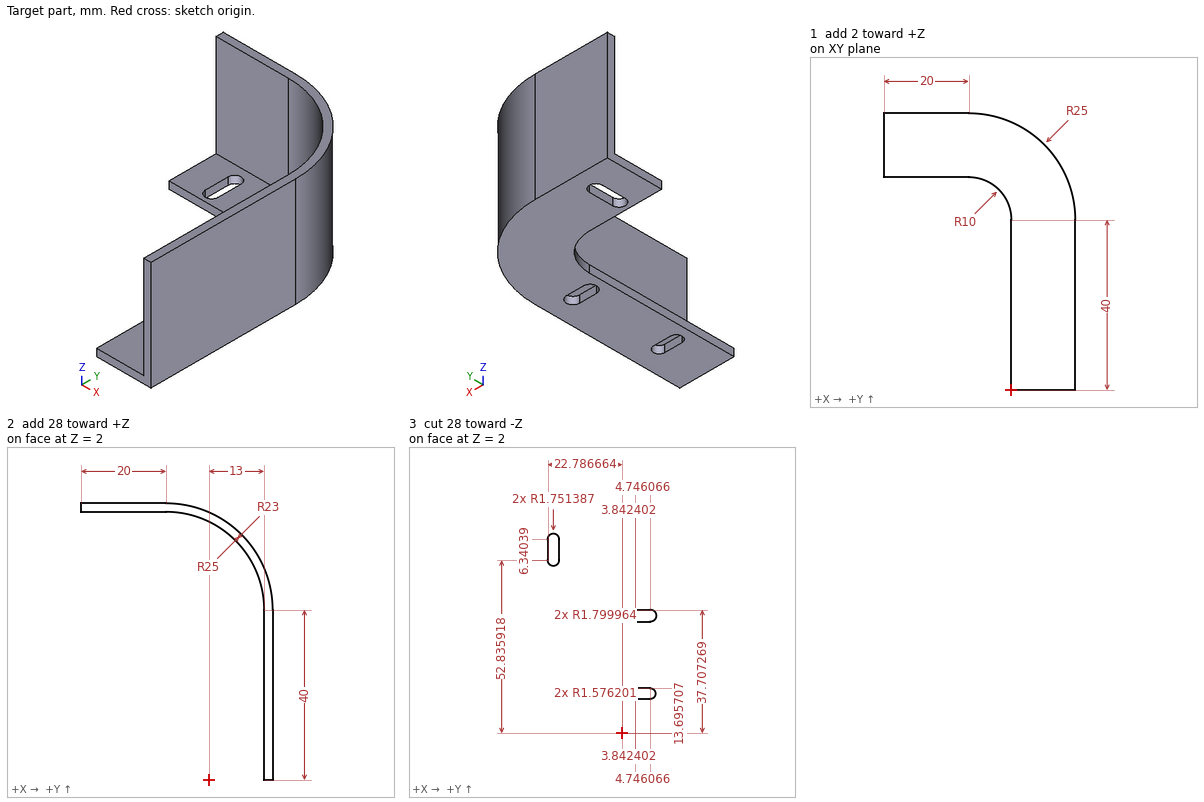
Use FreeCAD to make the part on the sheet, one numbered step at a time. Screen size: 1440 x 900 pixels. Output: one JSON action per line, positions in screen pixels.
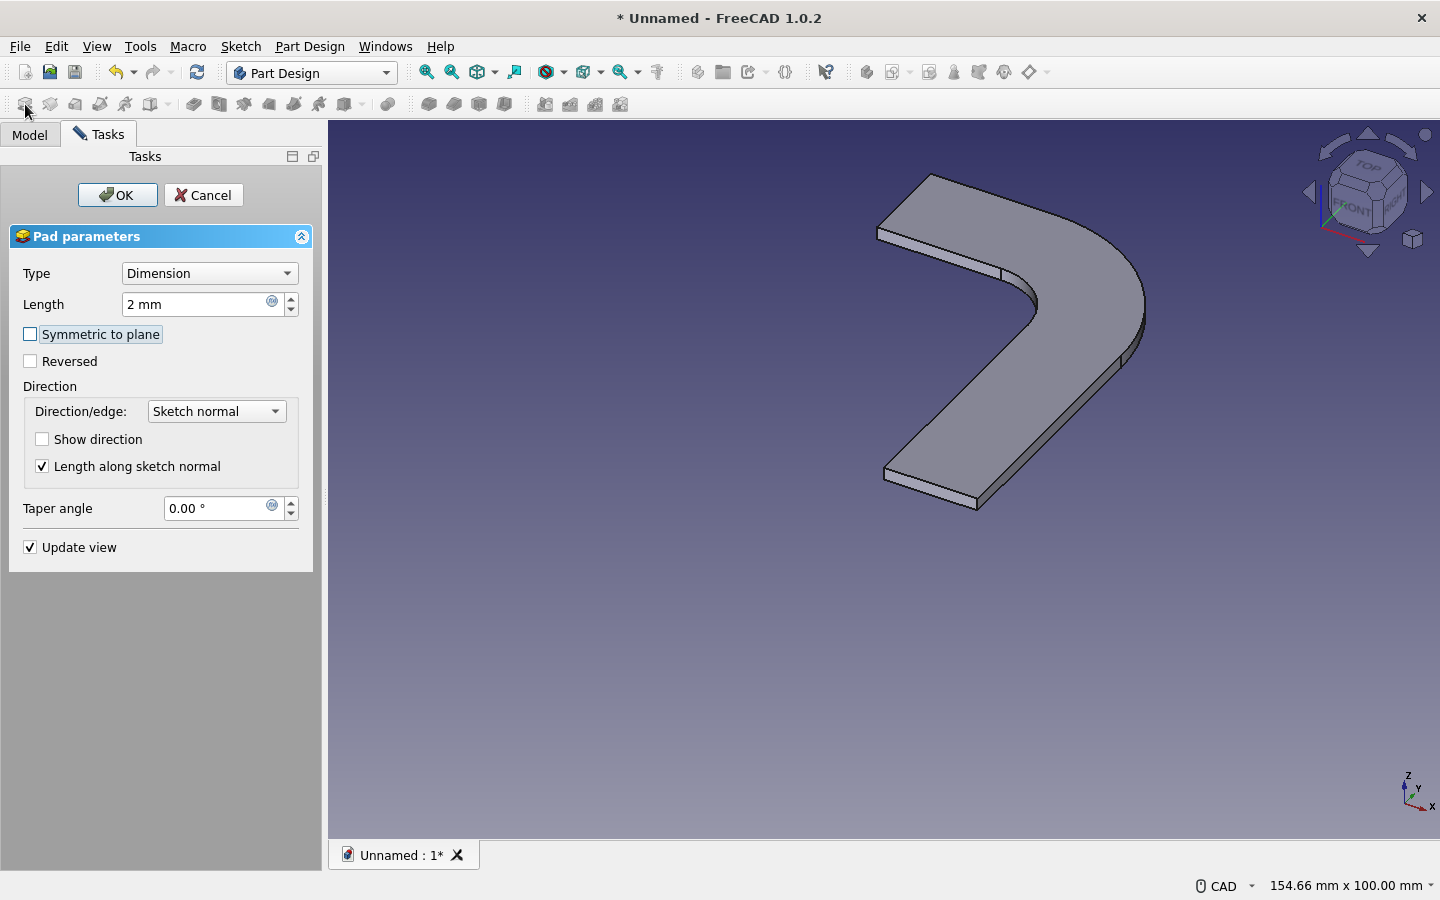
{"action": "left_click", "coordinate": [118, 195]}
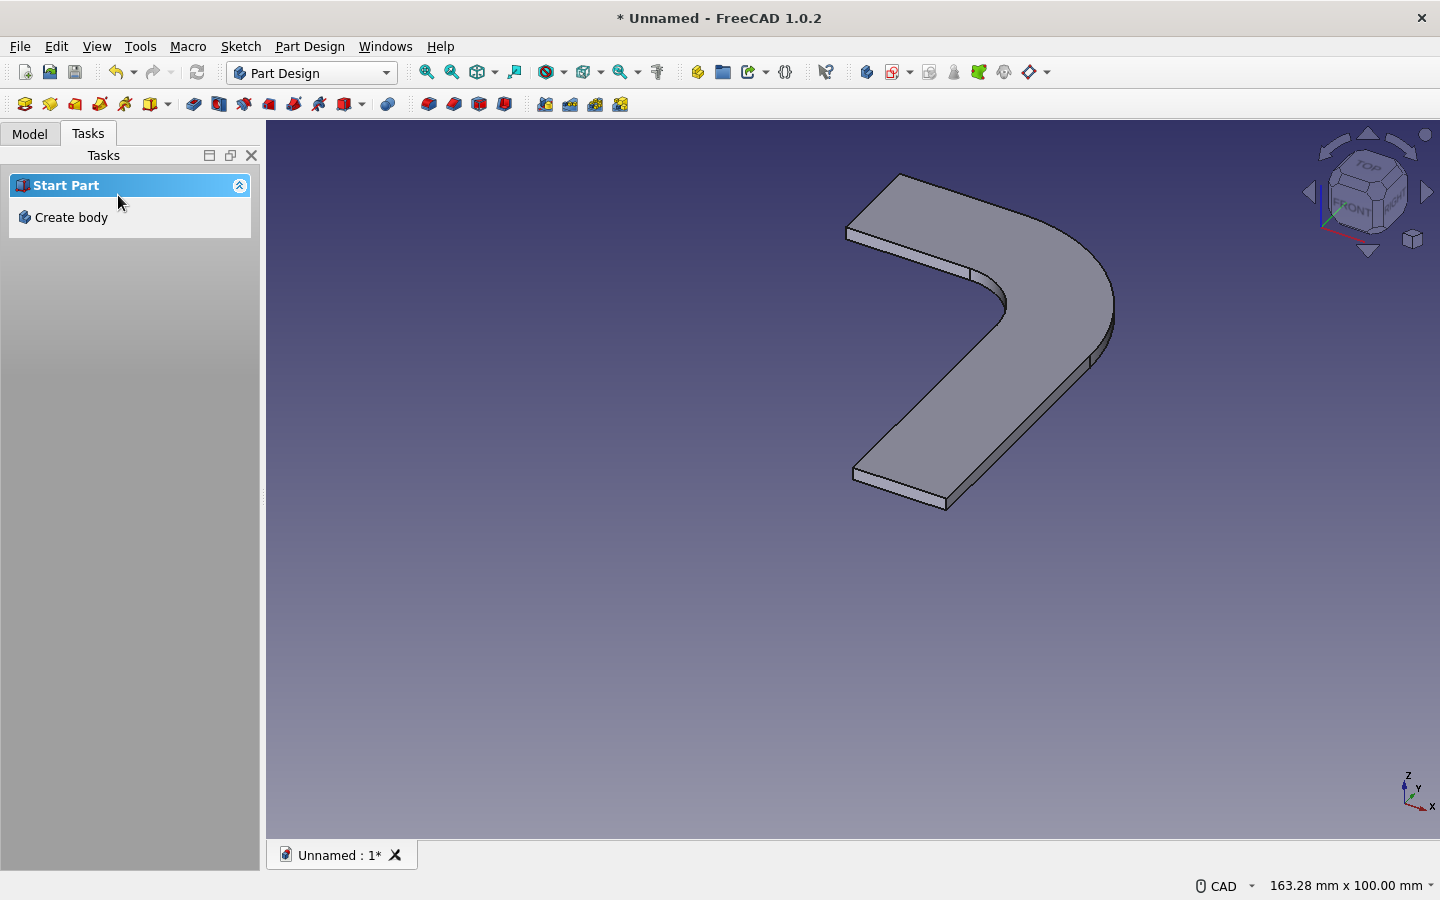
{"action": "left_click", "coordinate": [1070, 295]}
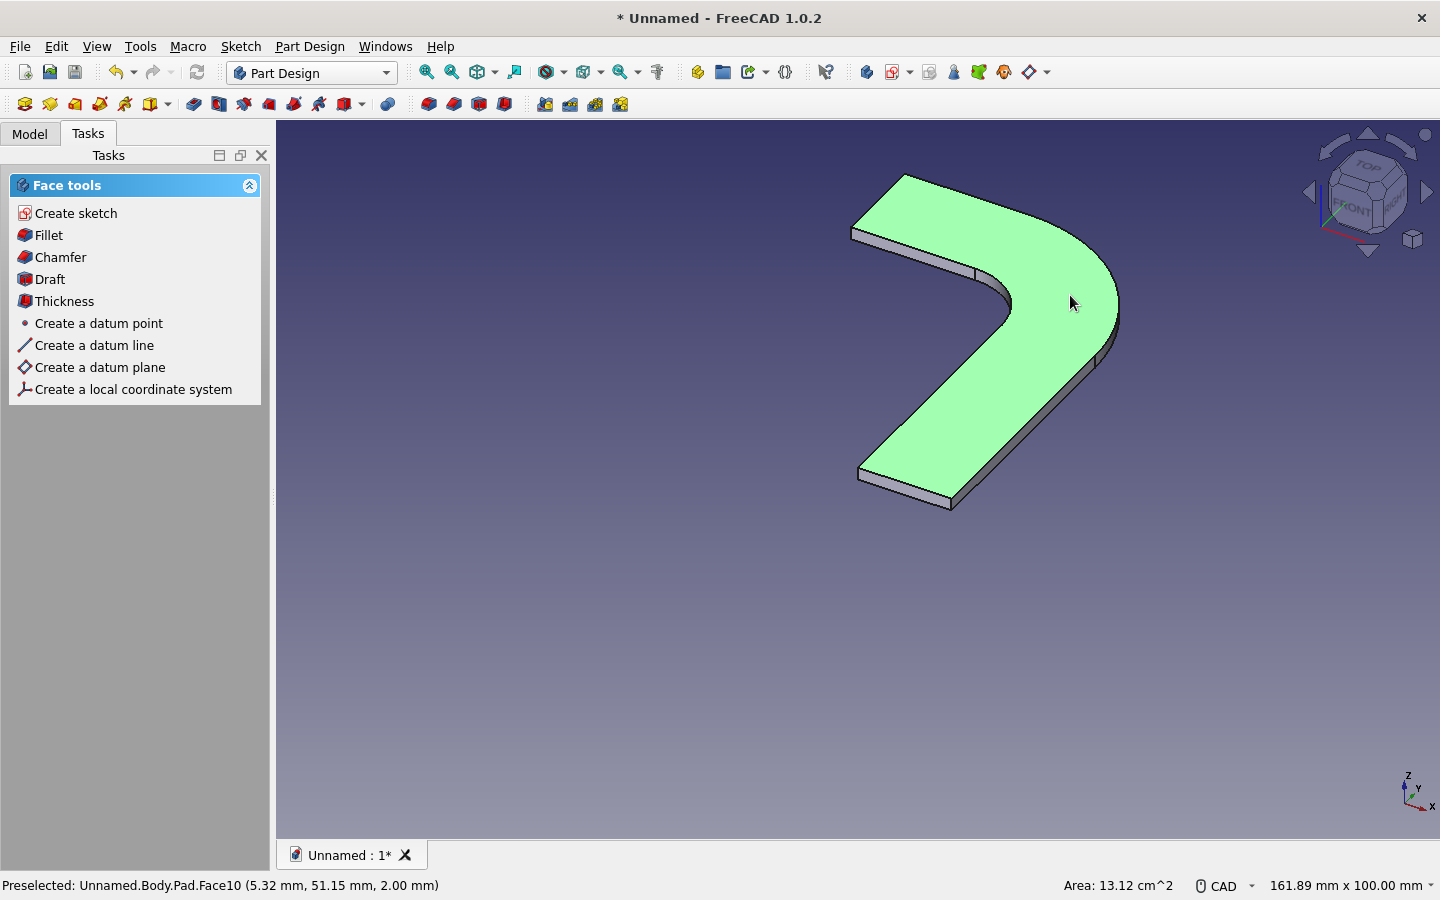
{"action": "left_click", "coordinate": [892, 72]}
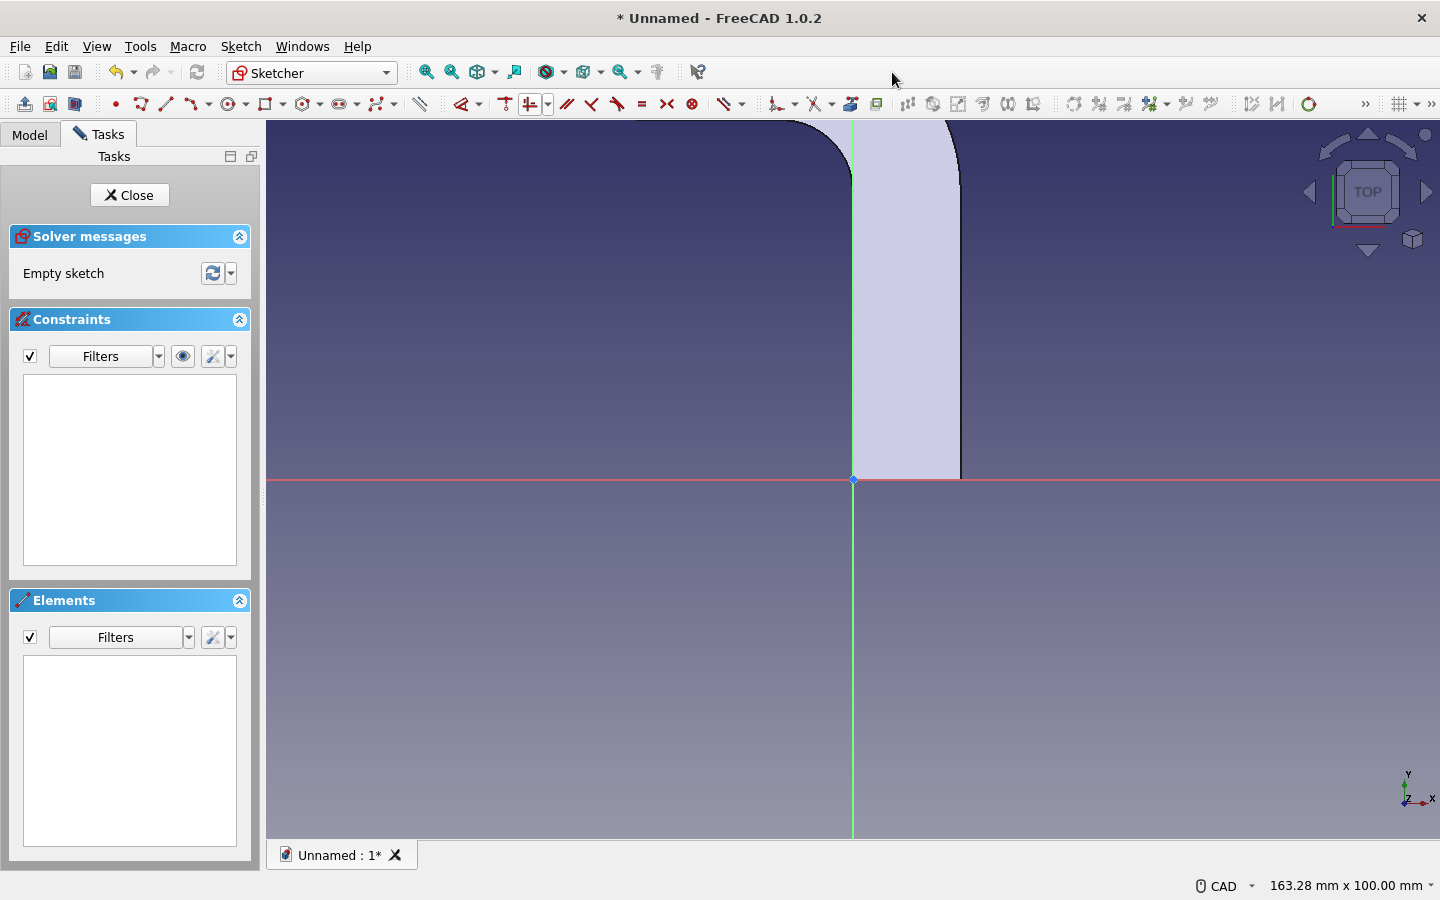
{"action": "scroll", "coordinate": [755, 811], "scroll_direction": "down", "scroll_amount": 2}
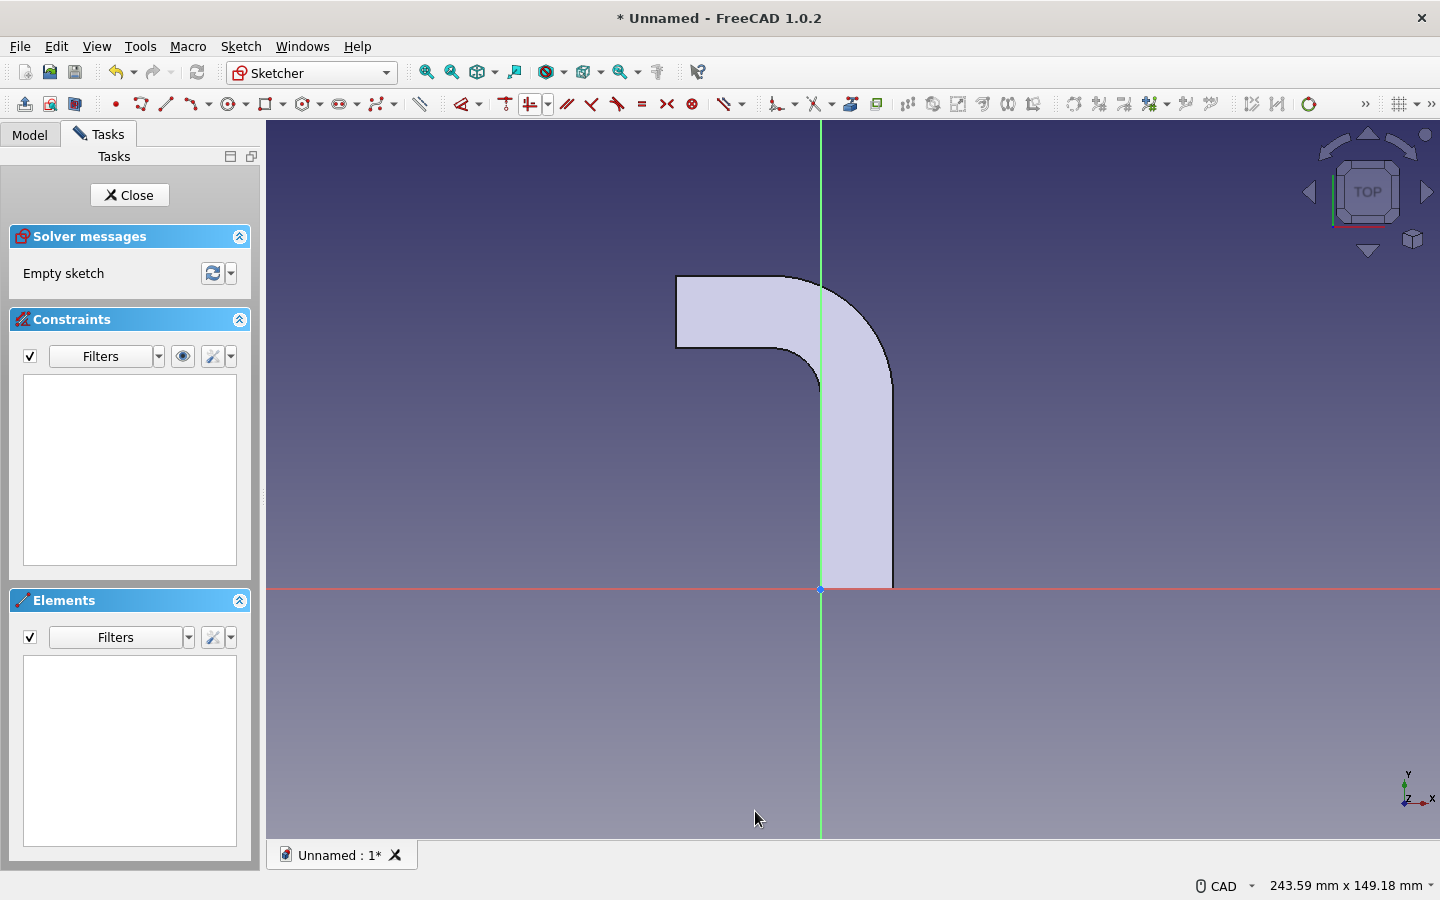
{"action": "scroll", "coordinate": [785, 337], "scroll_direction": "up", "scroll_amount": 2}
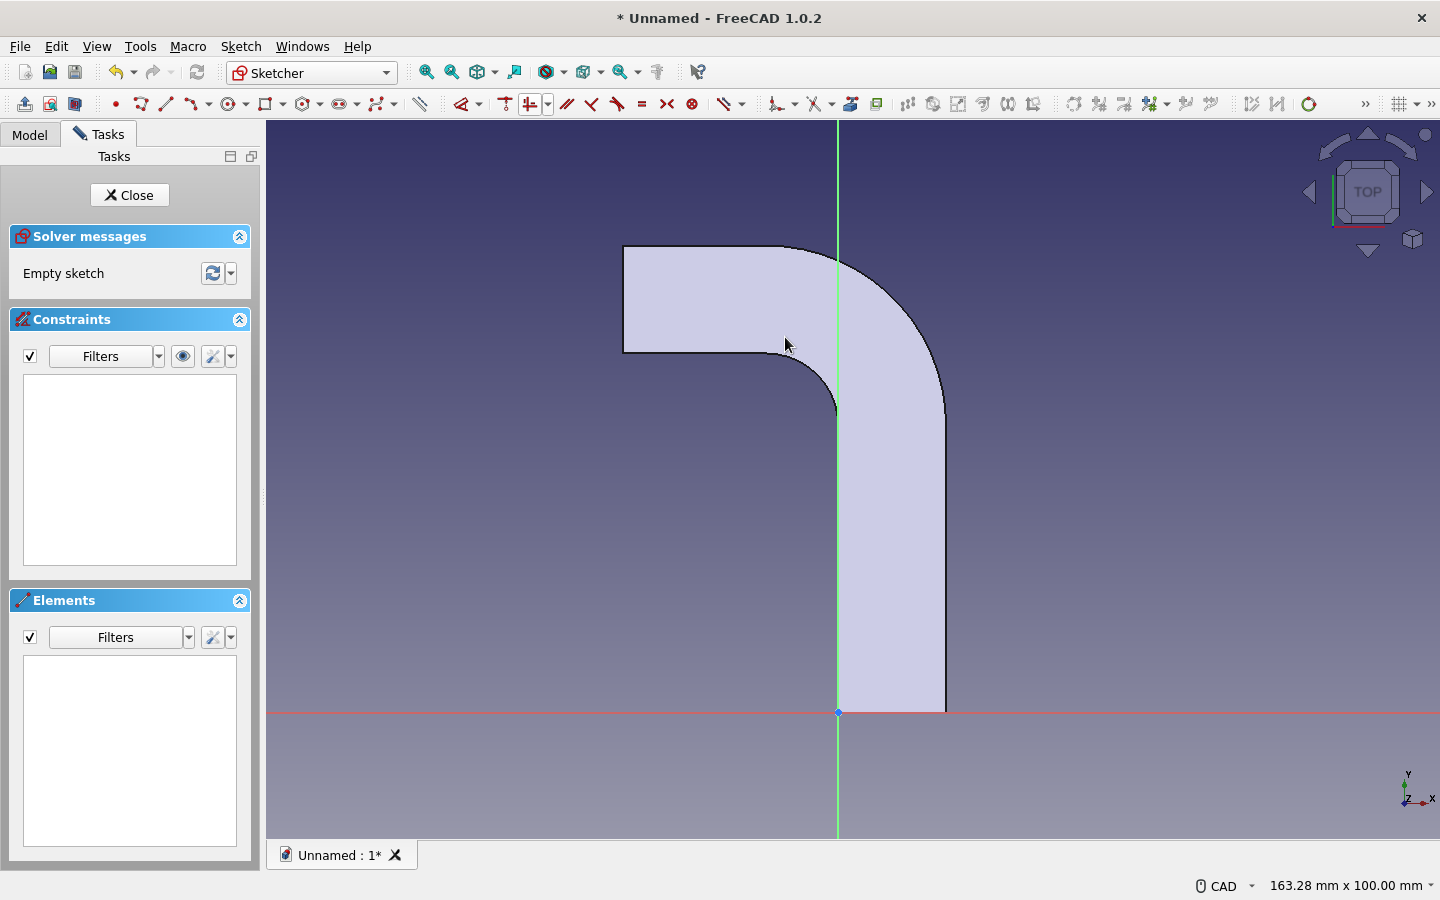
{"action": "left_click", "coordinate": [141, 104]}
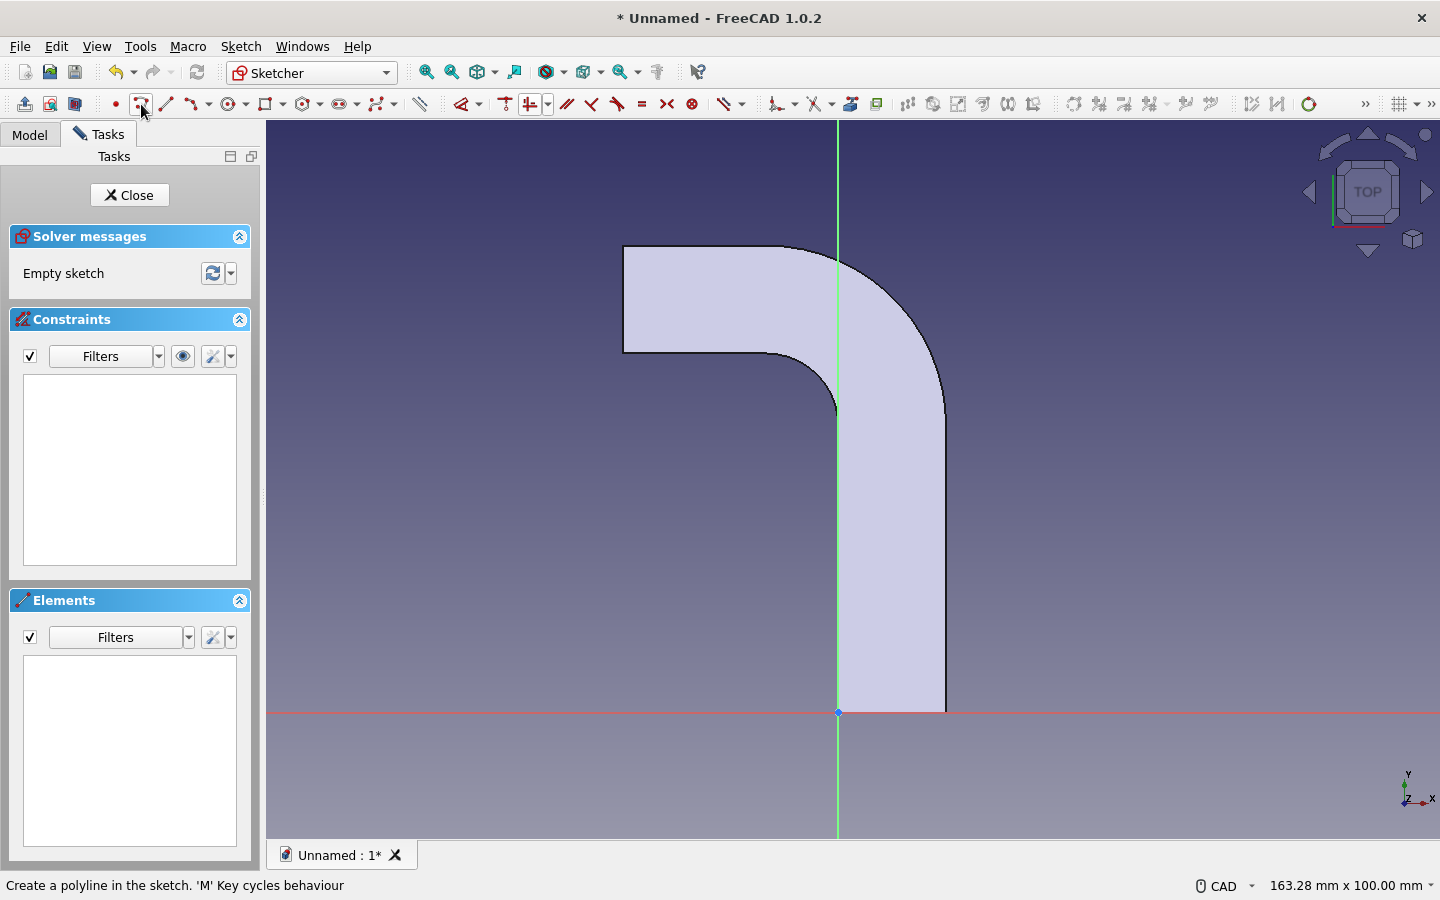
{"action": "left_click", "coordinate": [932, 425]}
{"action": "left_click", "coordinate": [932, 713]}
{"action": "left_click", "coordinate": [946, 704]}
{"action": "left_click", "coordinate": [946, 425]}
{"action": "right_click", "coordinate": [946, 425]}